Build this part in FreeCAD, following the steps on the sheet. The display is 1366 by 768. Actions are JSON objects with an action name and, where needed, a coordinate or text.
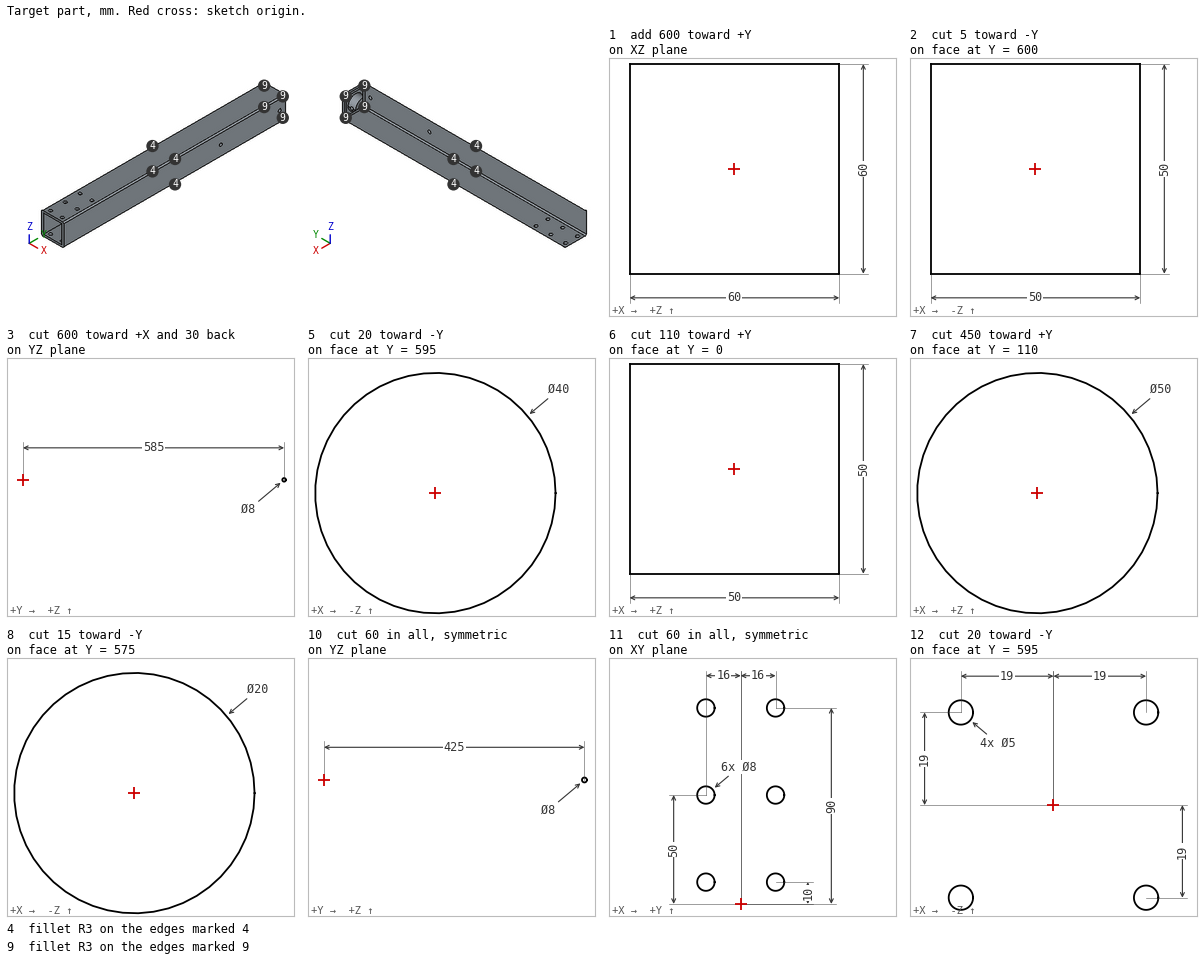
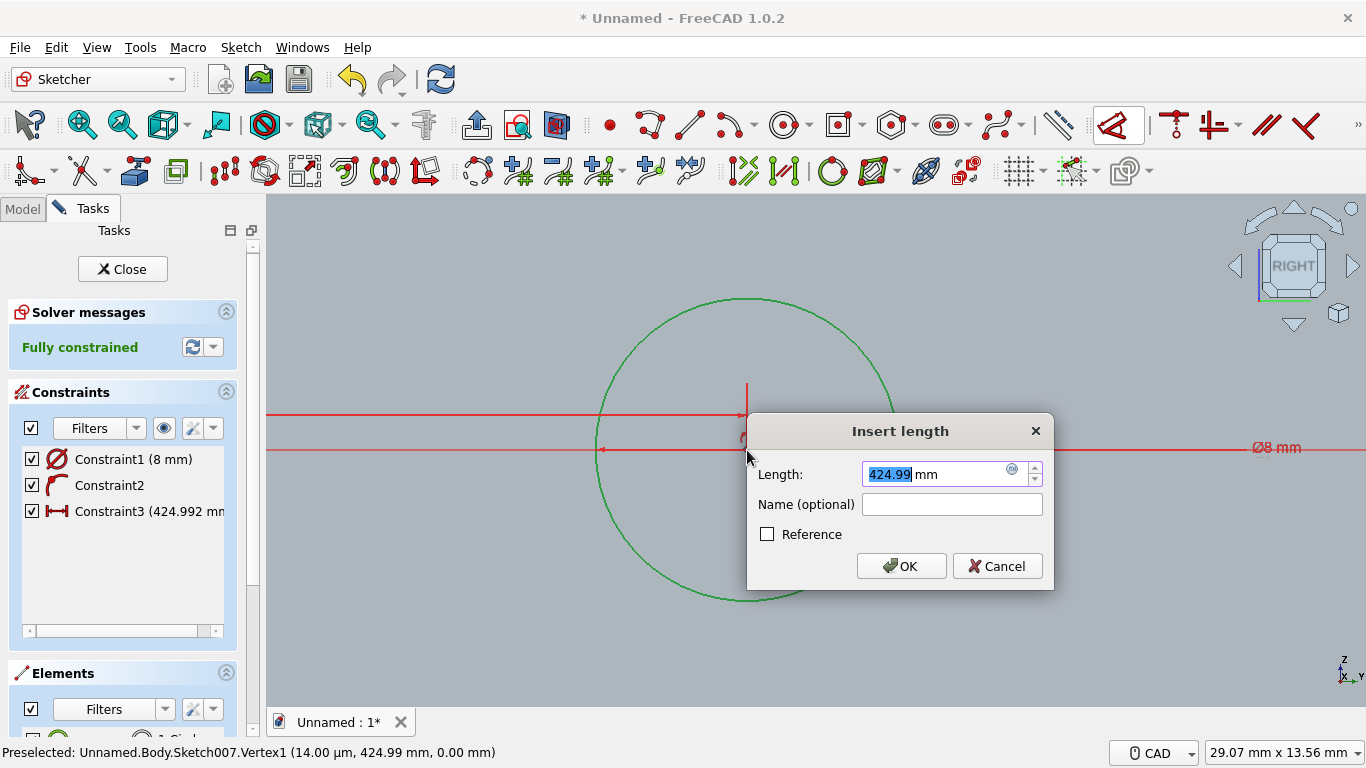
{"action": "type", "text": "425"}
{"action": "key", "text": "Return"}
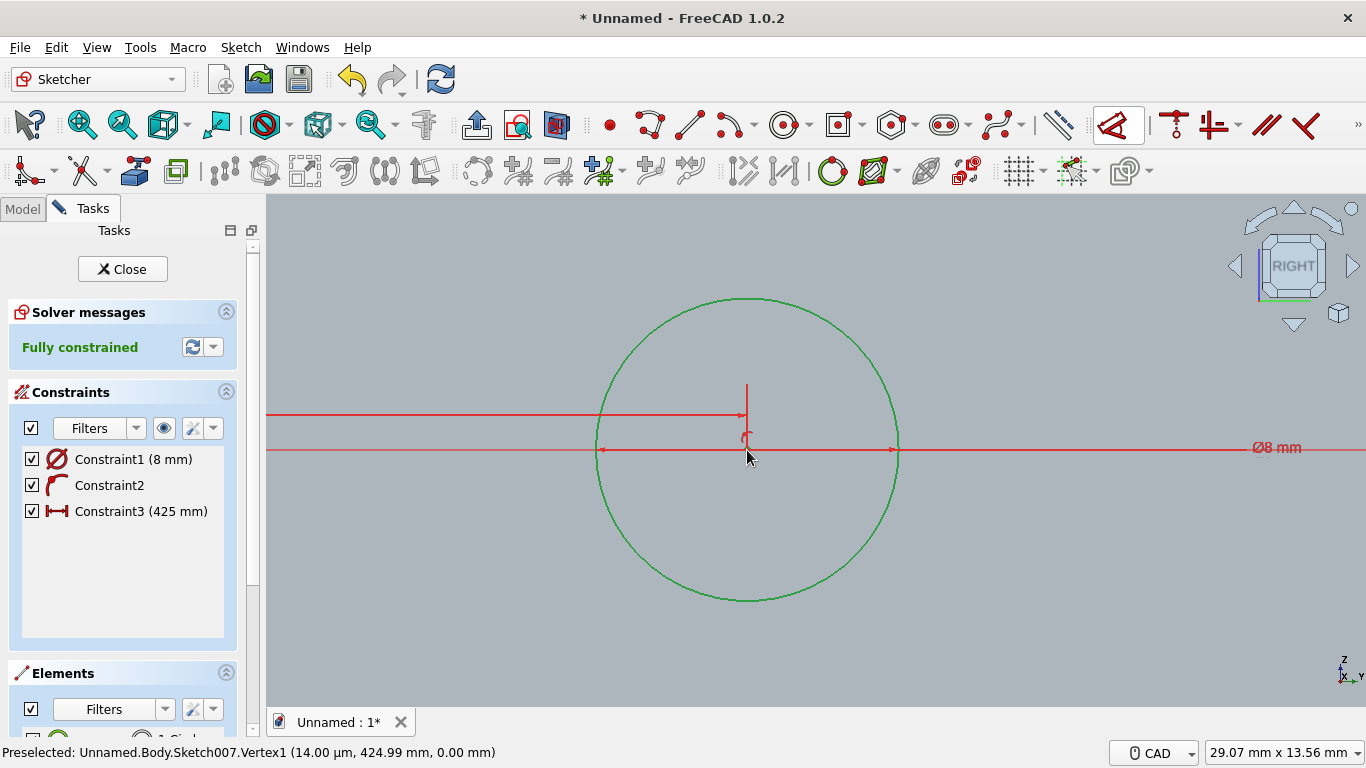
{"action": "left_click", "coordinate": [123, 269]}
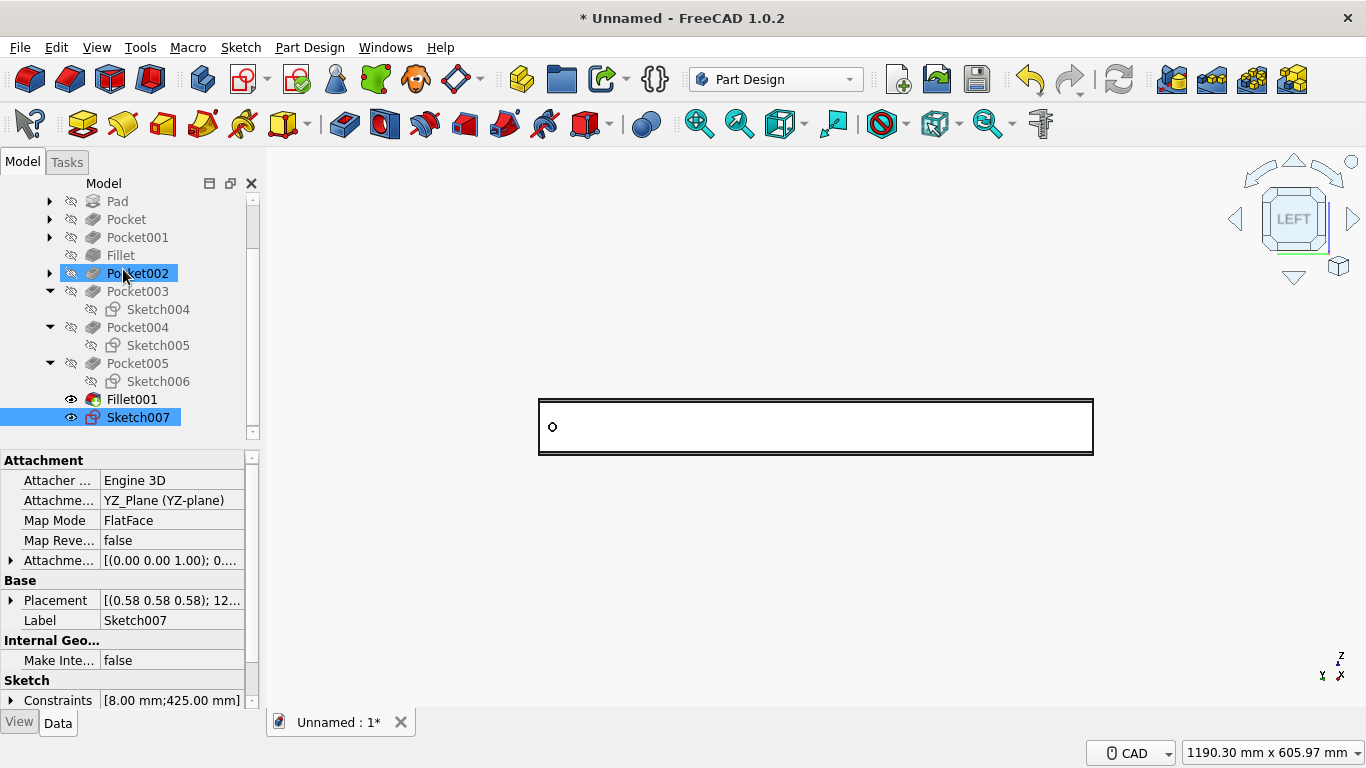
{"action": "left_click", "coordinate": [346, 124]}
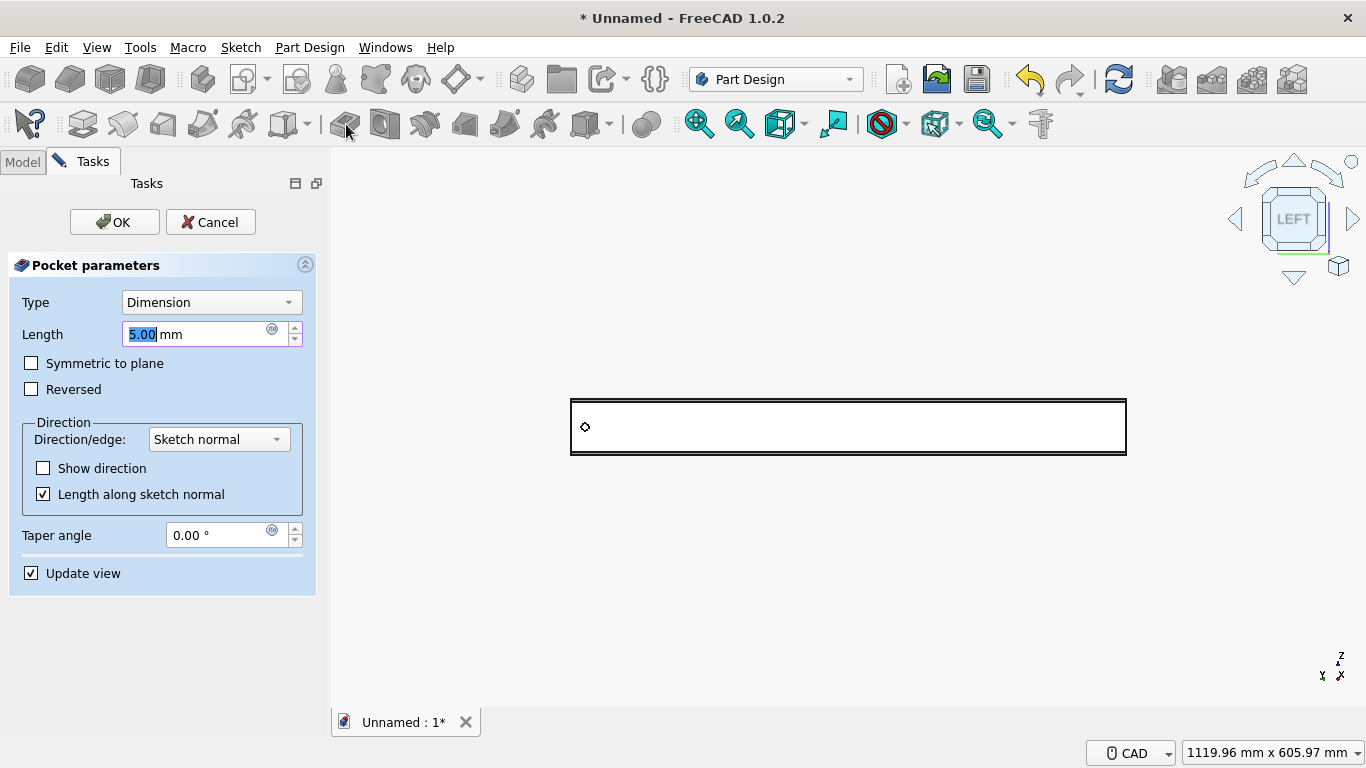
{"action": "type", "text": "60"}
{"action": "key", "text": "Tab"}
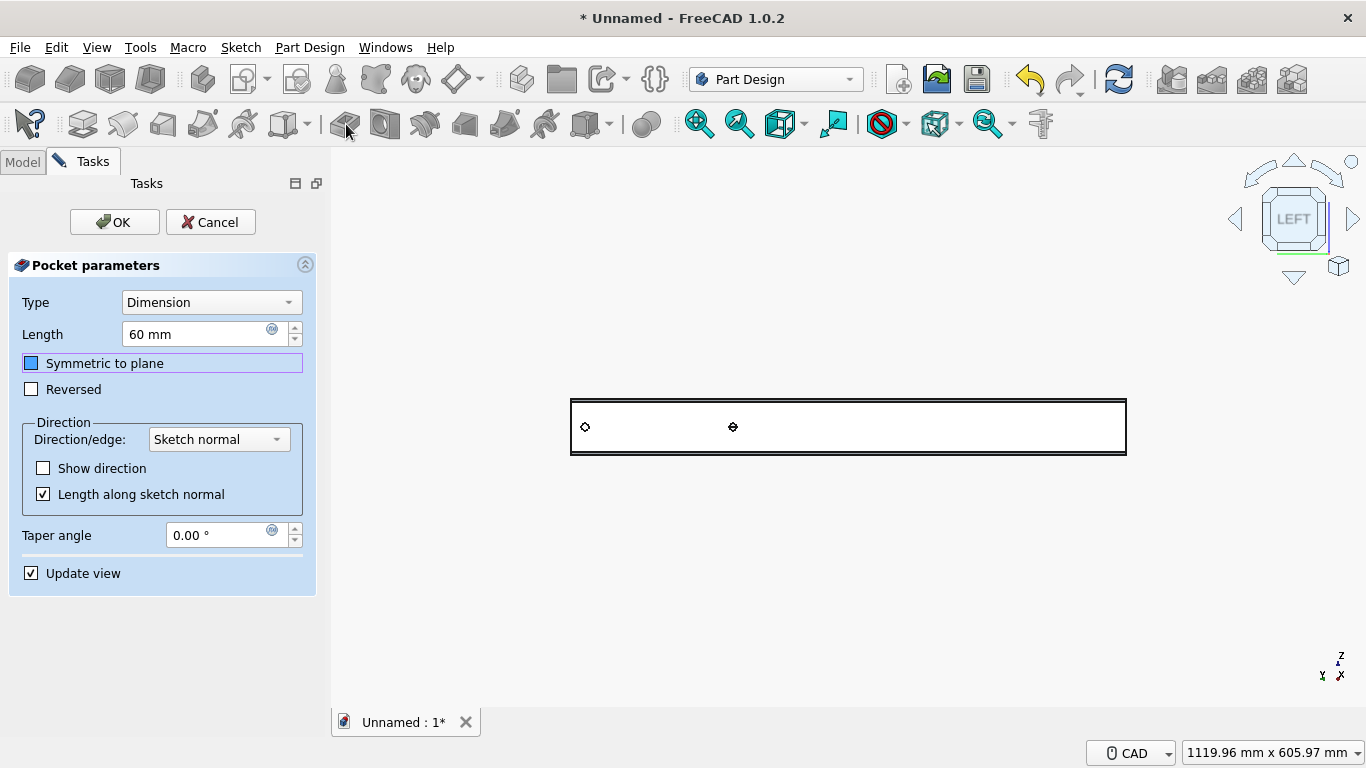
{"action": "left_click", "coordinate": [30, 363]}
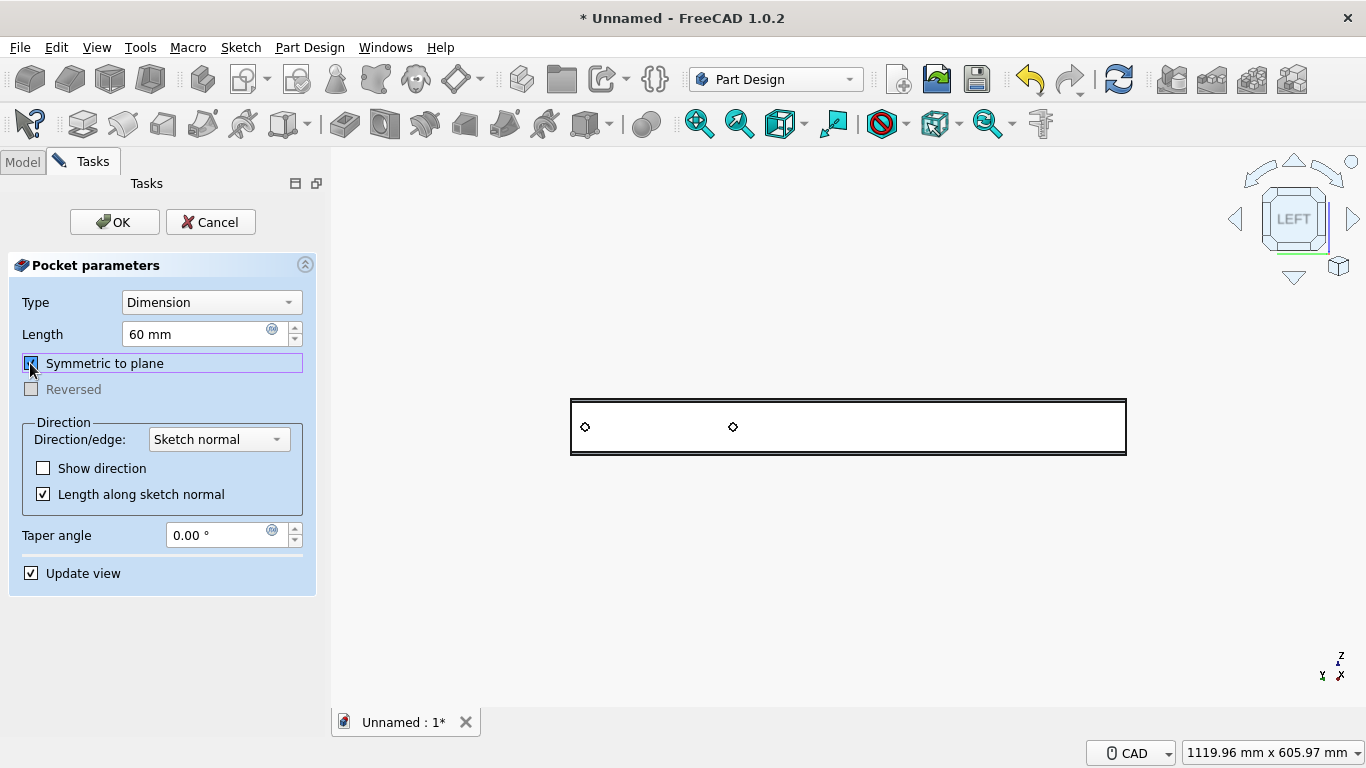
{"action": "left_click", "coordinate": [115, 222]}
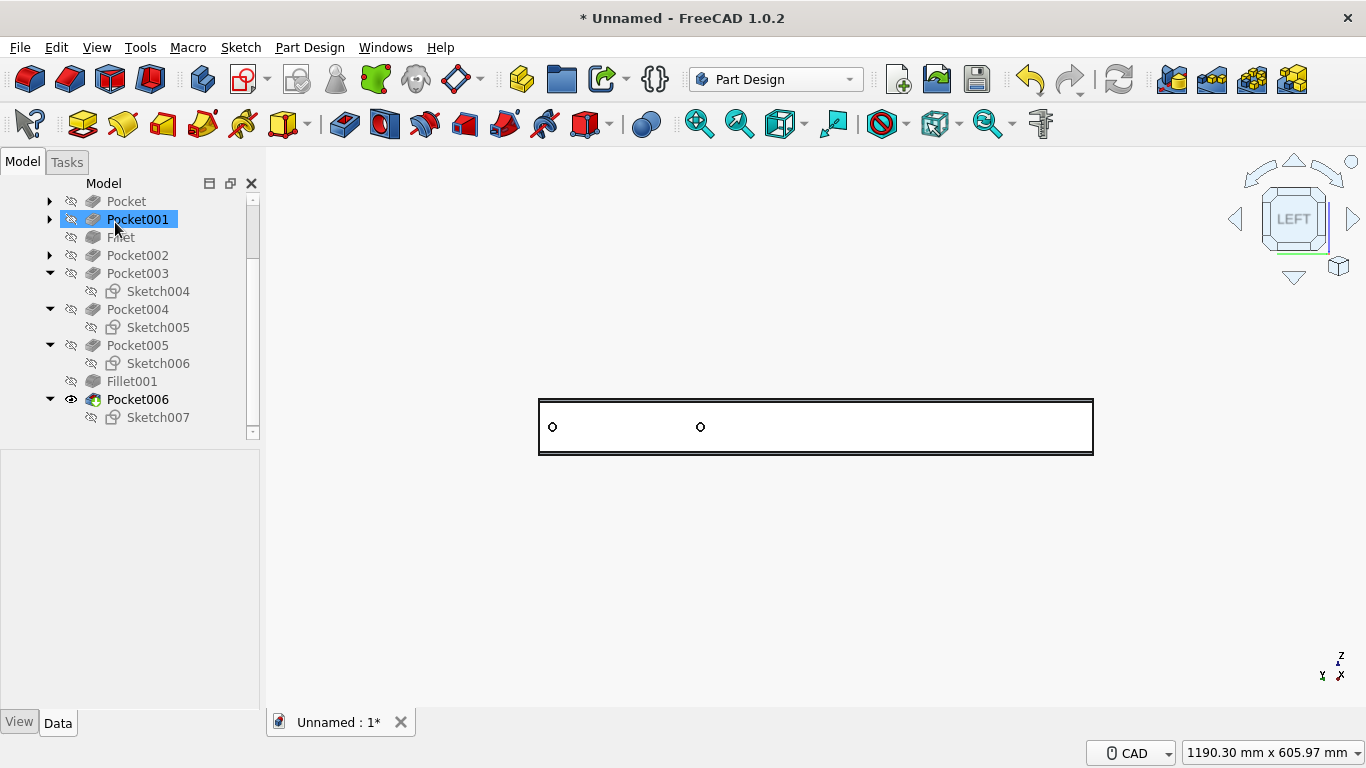
{"action": "left_click", "coordinate": [244, 80]}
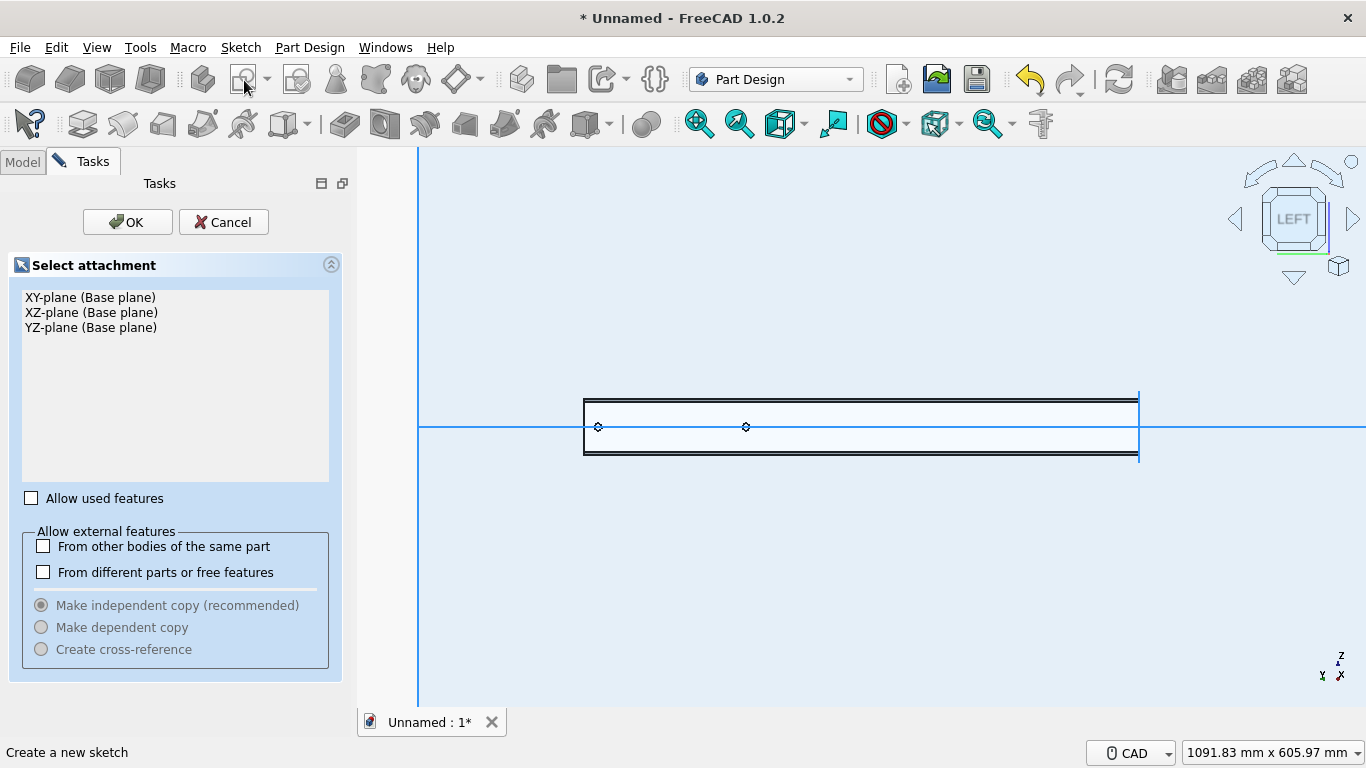
{"action": "left_click", "coordinate": [82, 298]}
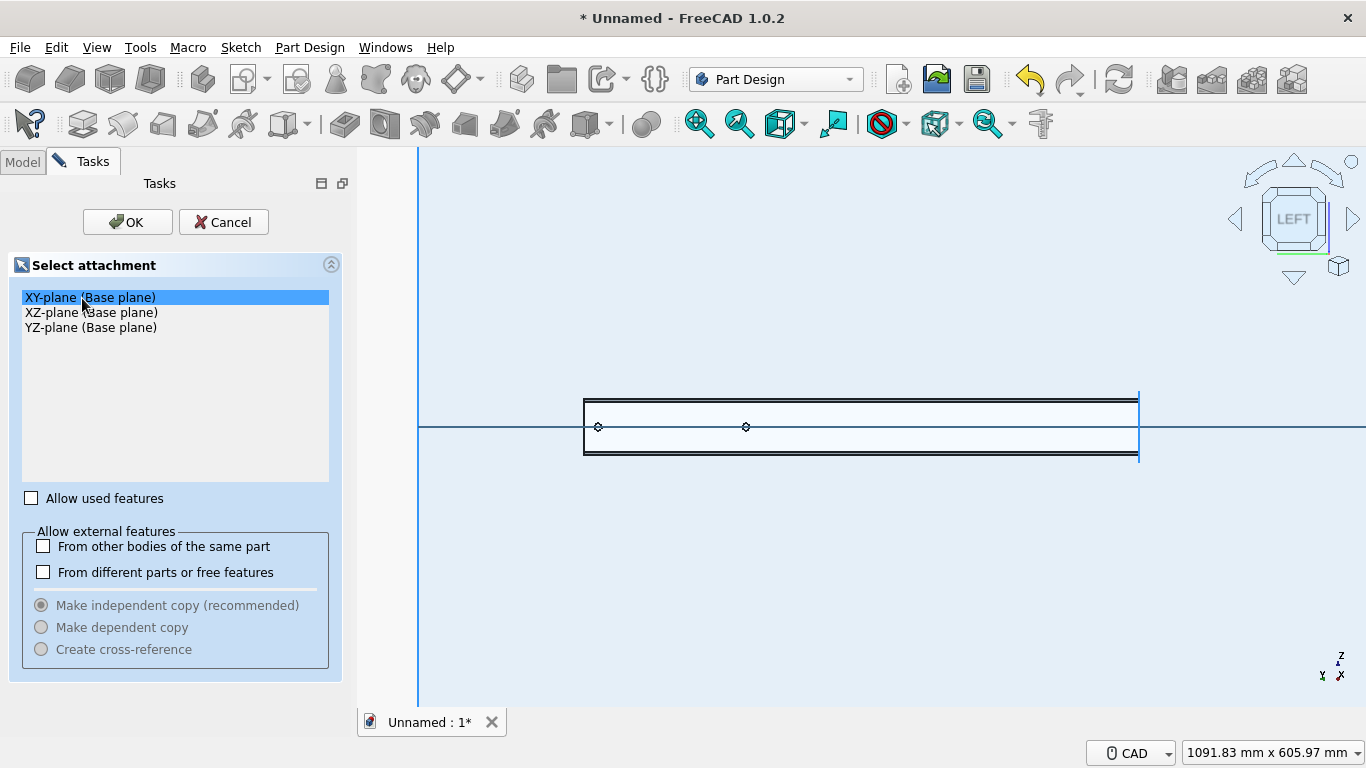
{"action": "left_click", "coordinate": [128, 222]}